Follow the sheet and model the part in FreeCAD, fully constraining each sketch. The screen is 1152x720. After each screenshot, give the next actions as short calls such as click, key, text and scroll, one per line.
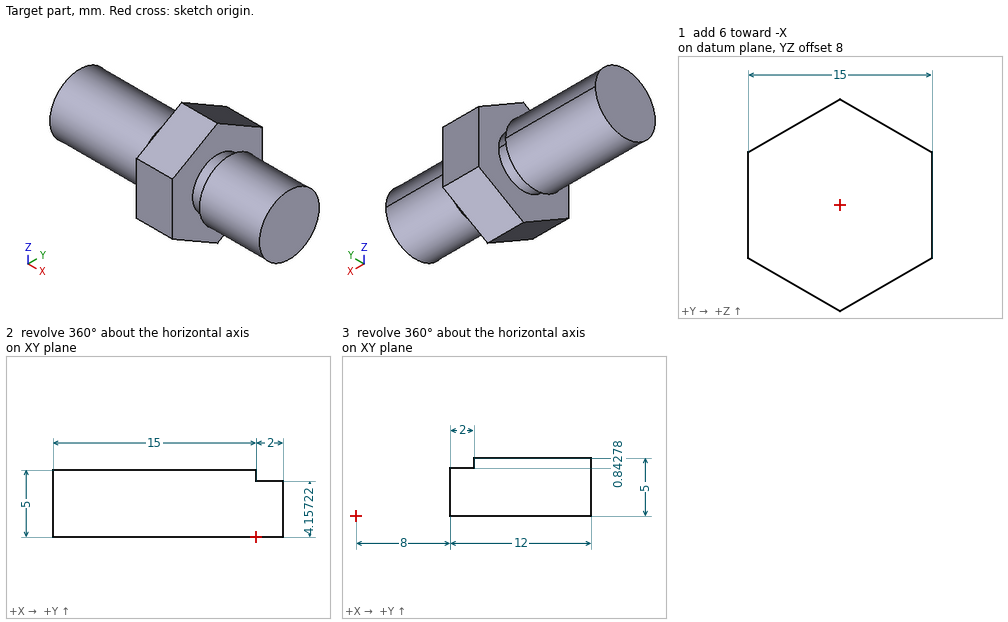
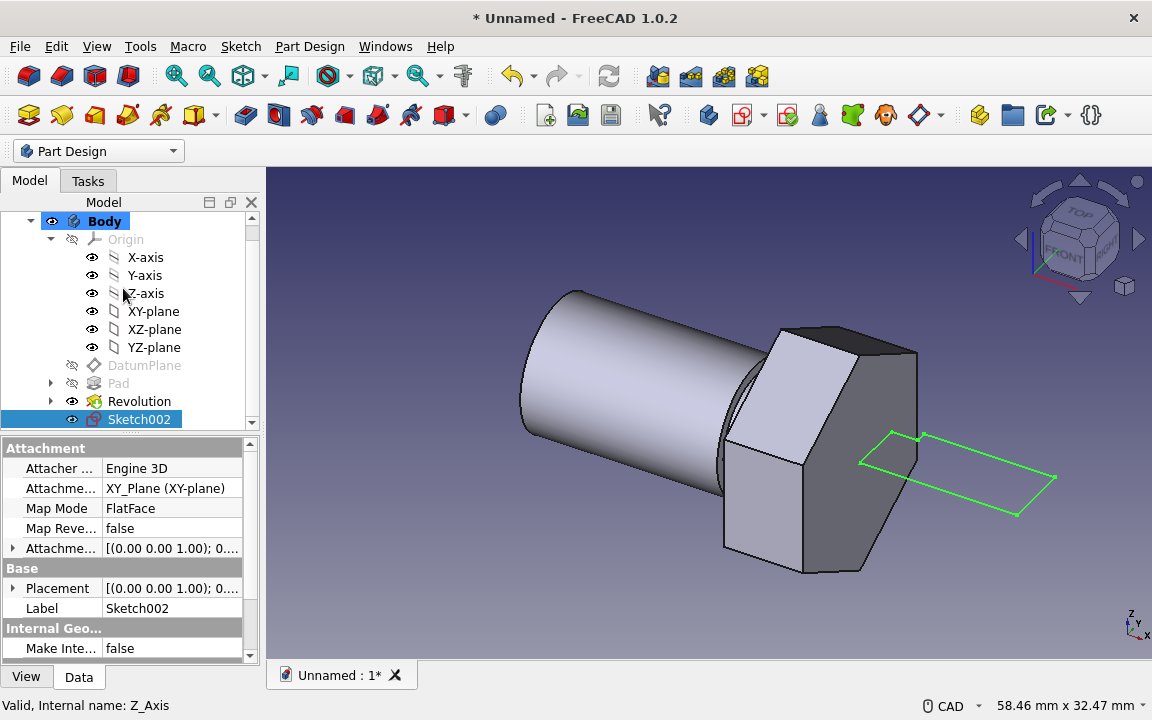
click(62, 116)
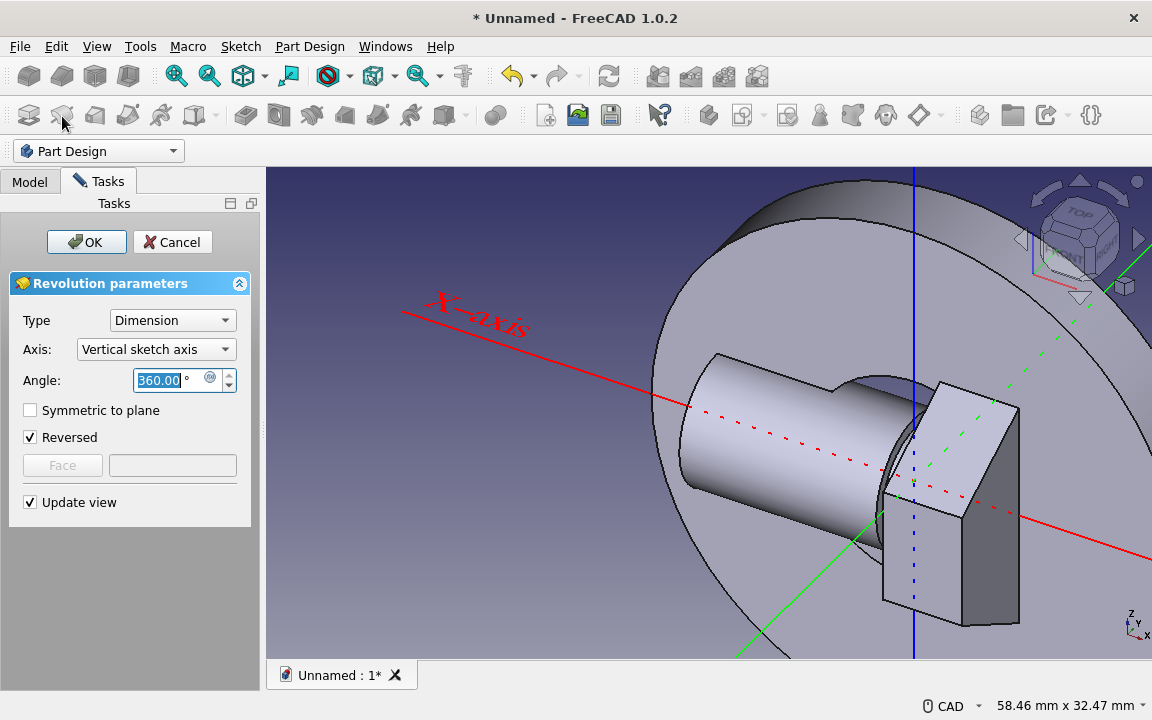
click(157, 350)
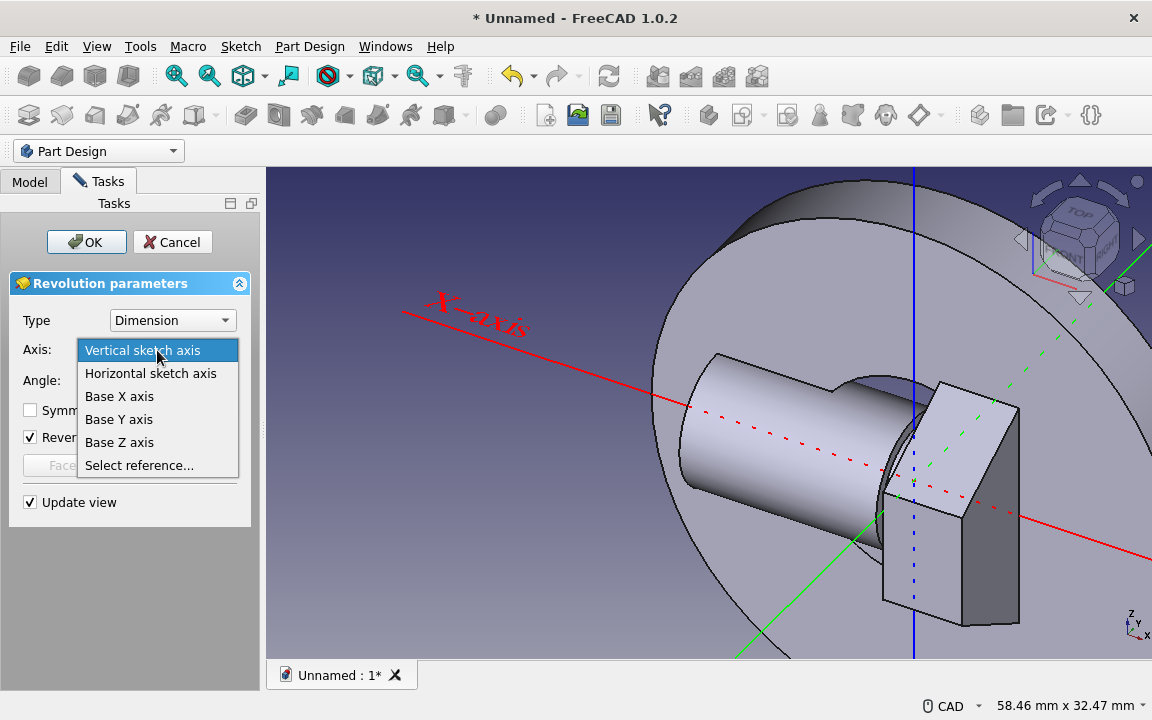
click(156, 374)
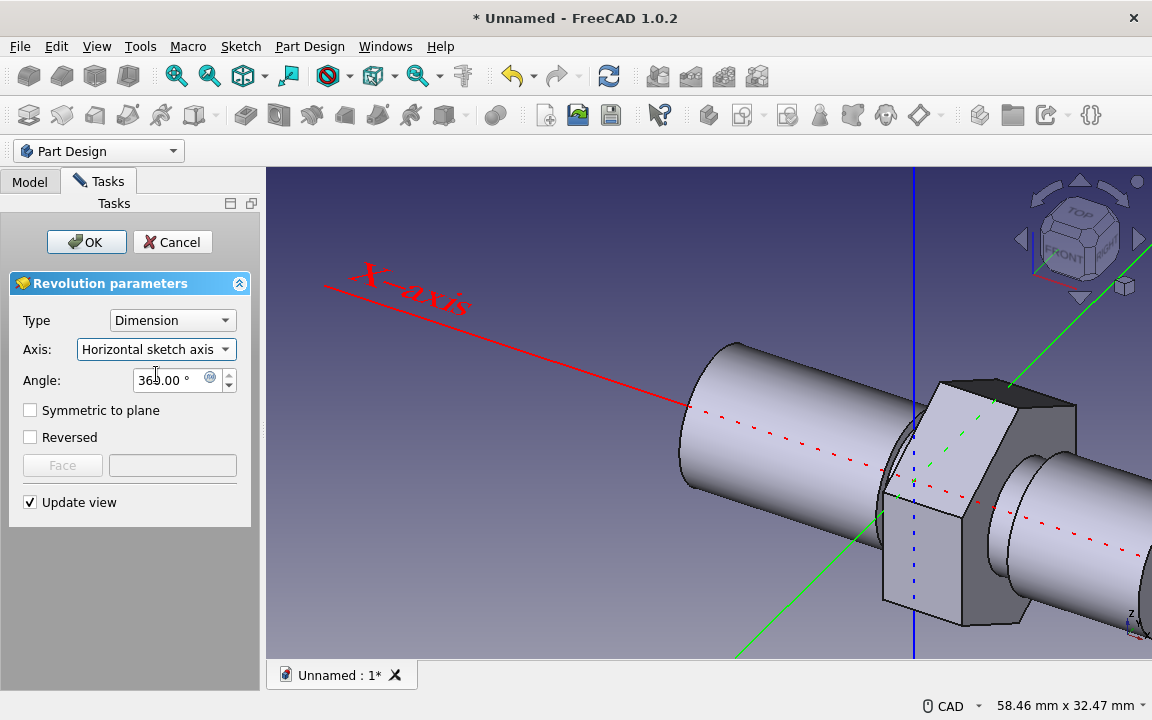
click(87, 242)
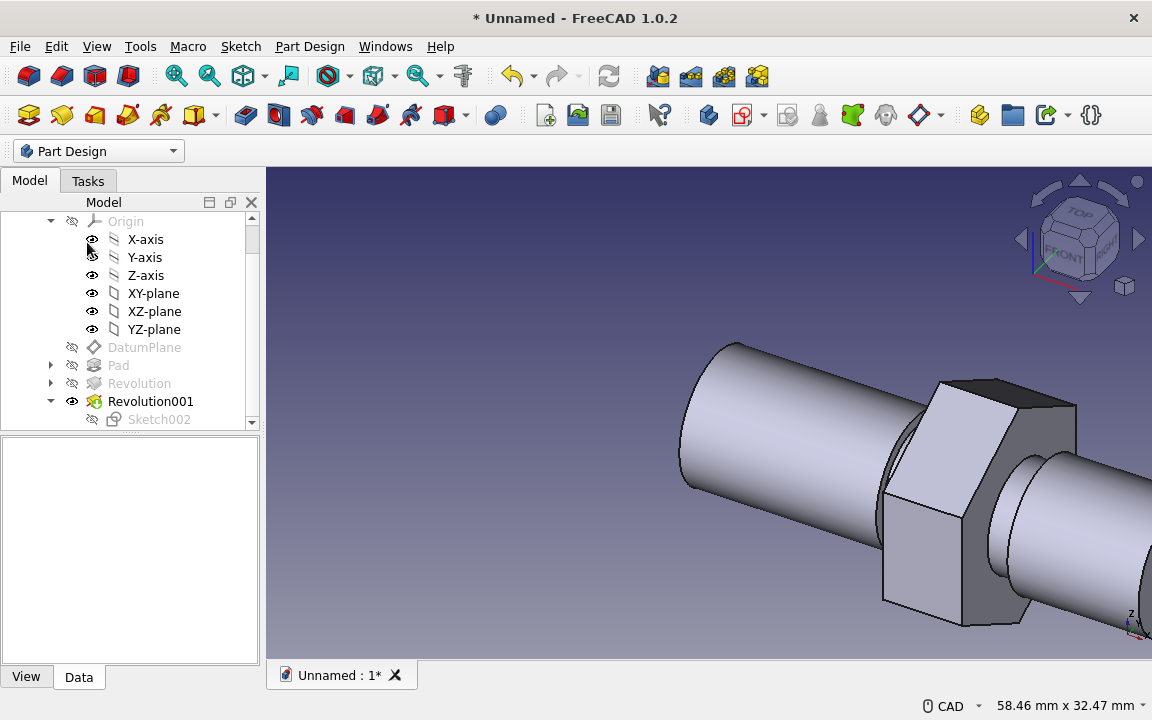
key(0)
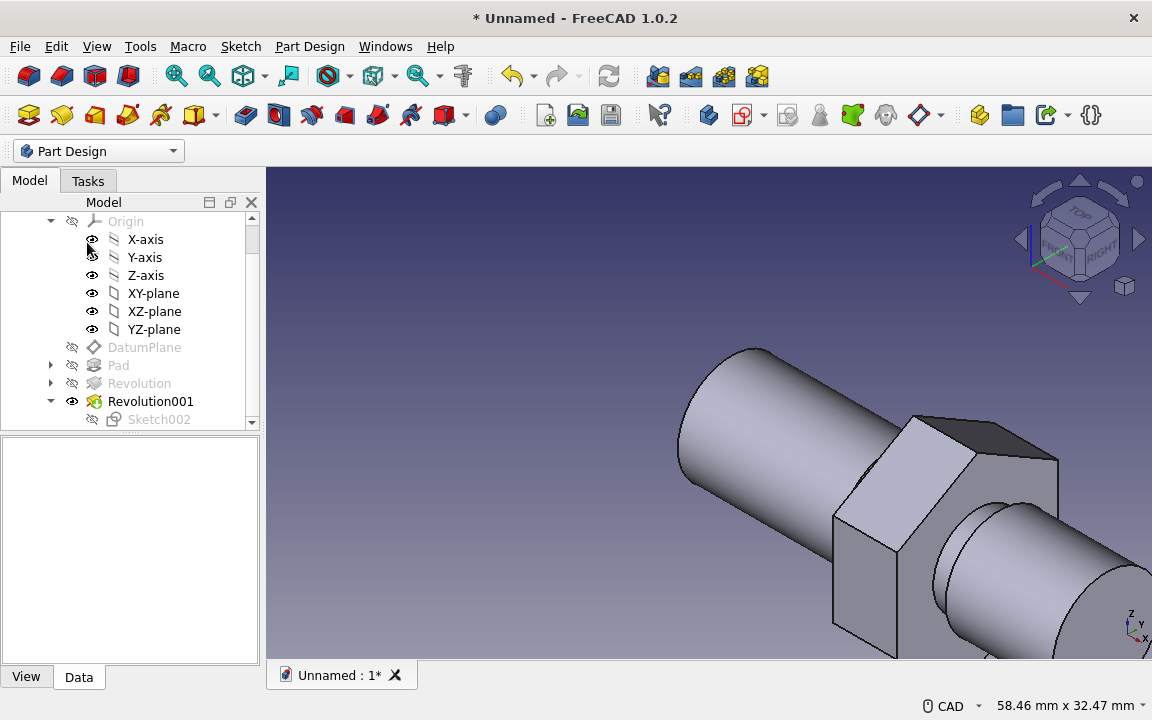
key(v)
key(f)